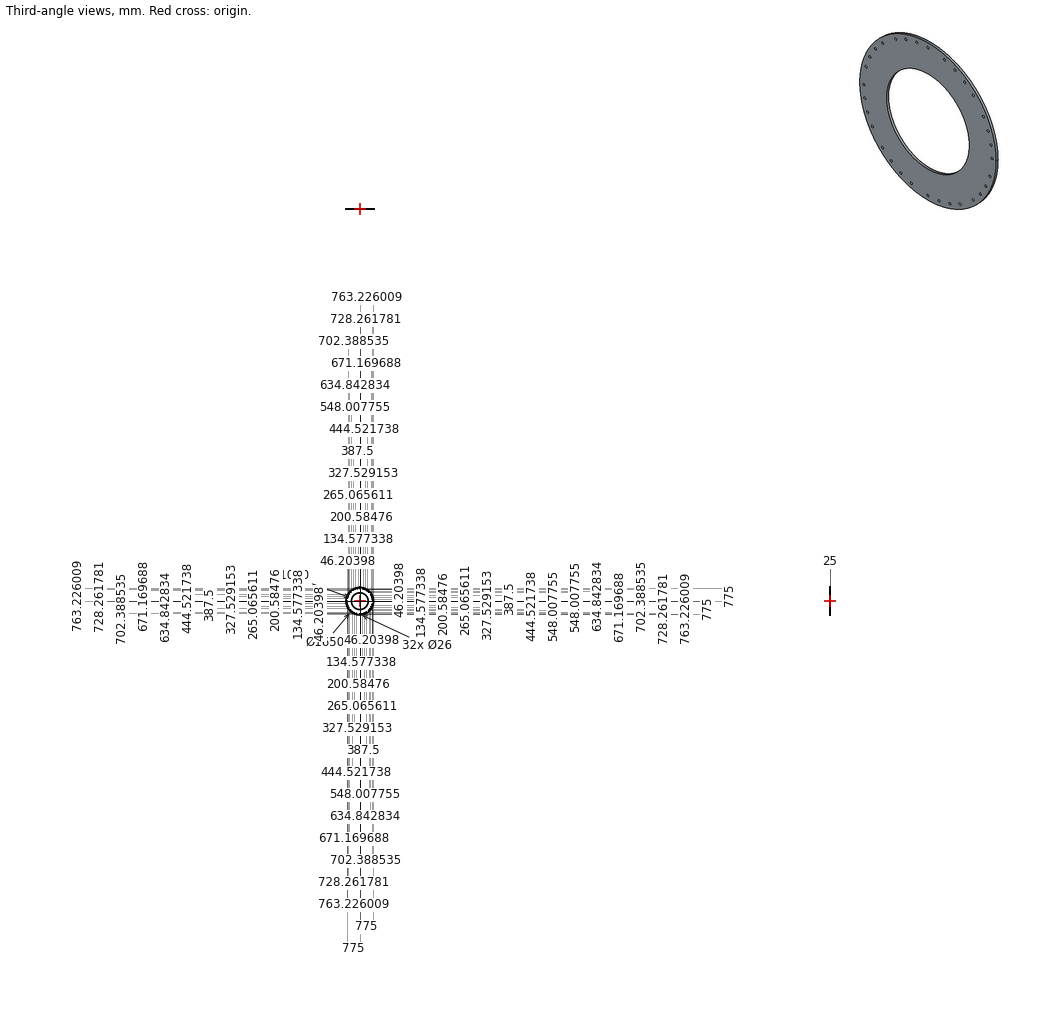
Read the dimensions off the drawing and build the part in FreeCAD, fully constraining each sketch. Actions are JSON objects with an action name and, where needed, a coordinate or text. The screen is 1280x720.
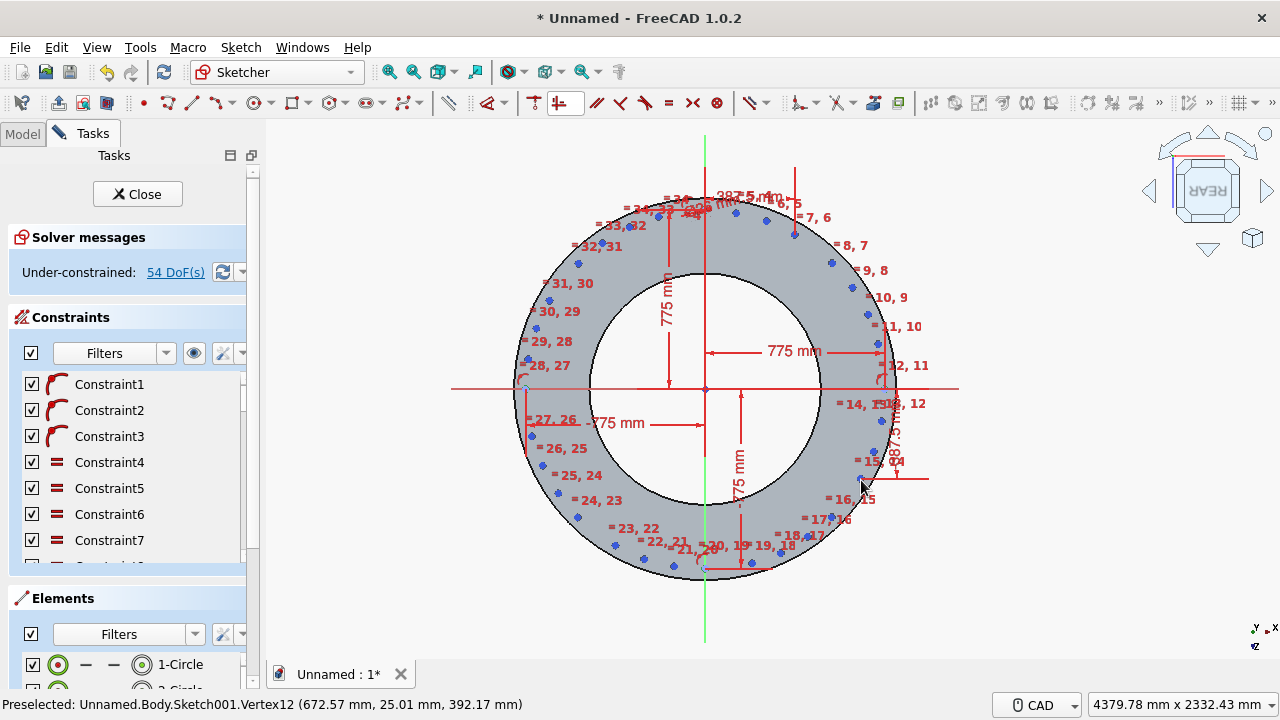
{"action": "left_click", "coordinate": [615, 546]}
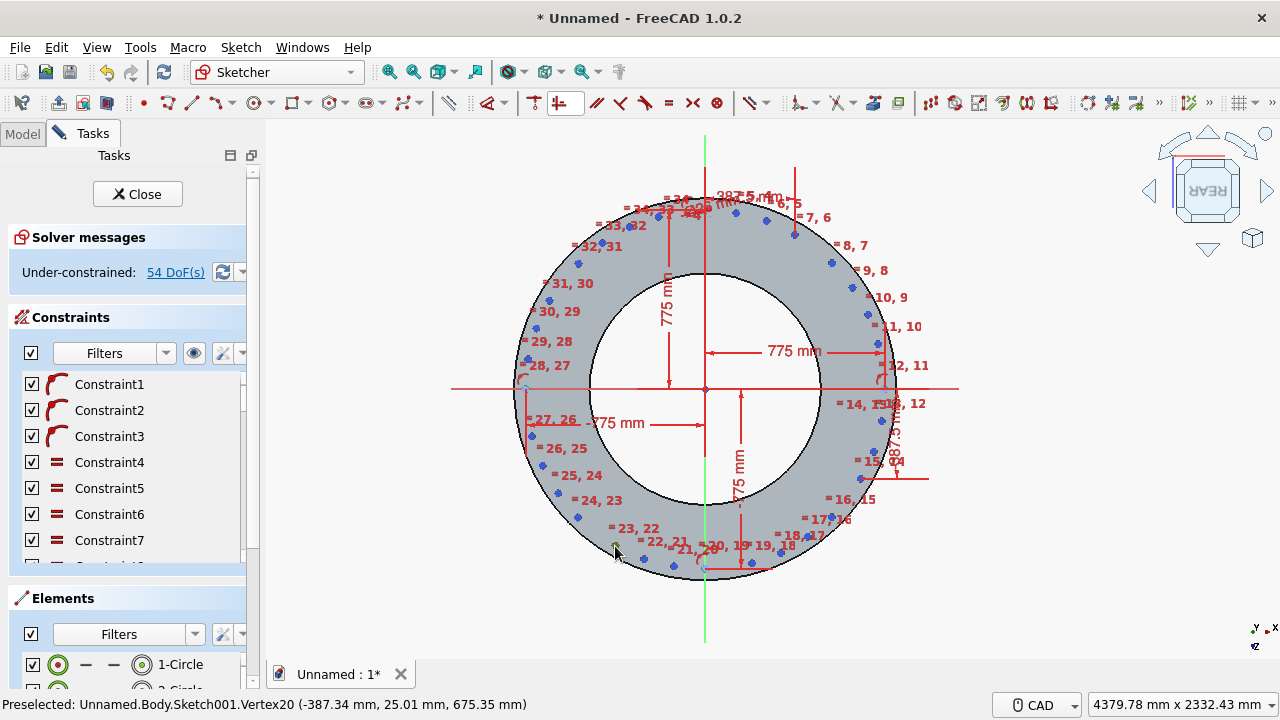
{"action": "left_click", "coordinate": [506, 104]}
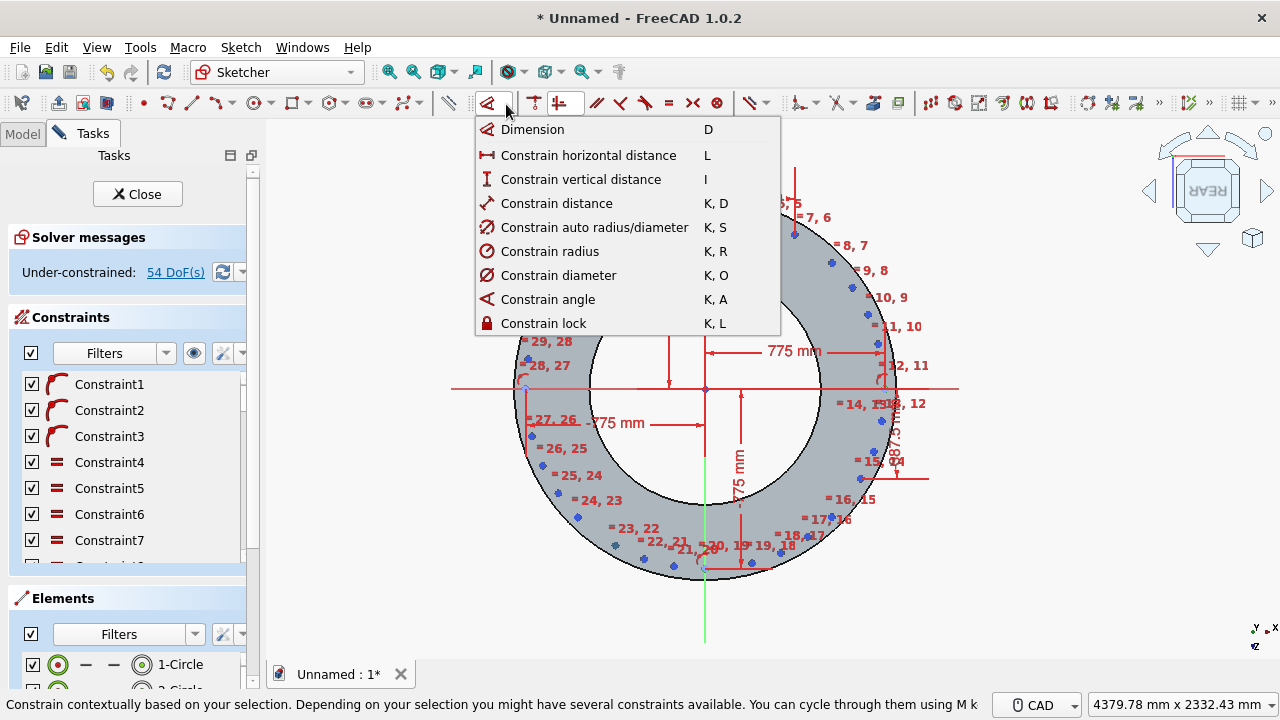
{"action": "left_click", "coordinate": [628, 155]}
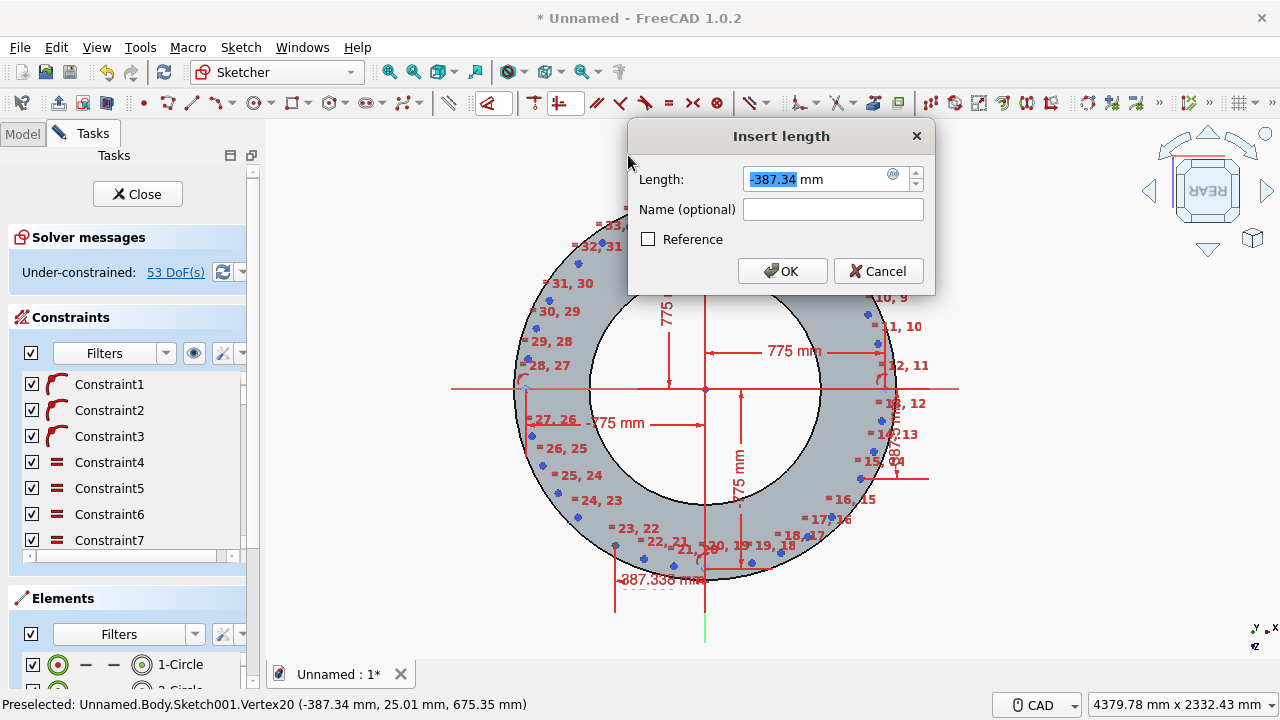
{"action": "type", "text": "-387.5"}
{"action": "key", "text": "Return"}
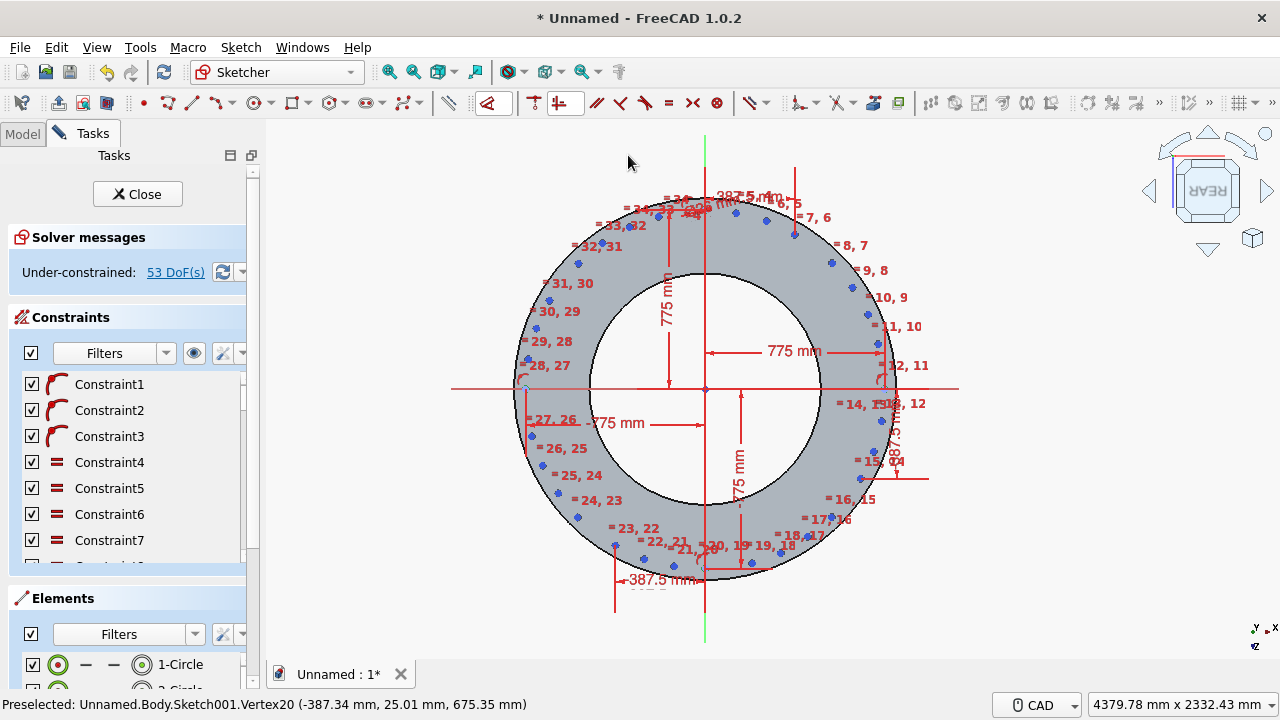
{"action": "left_click", "coordinate": [550, 301]}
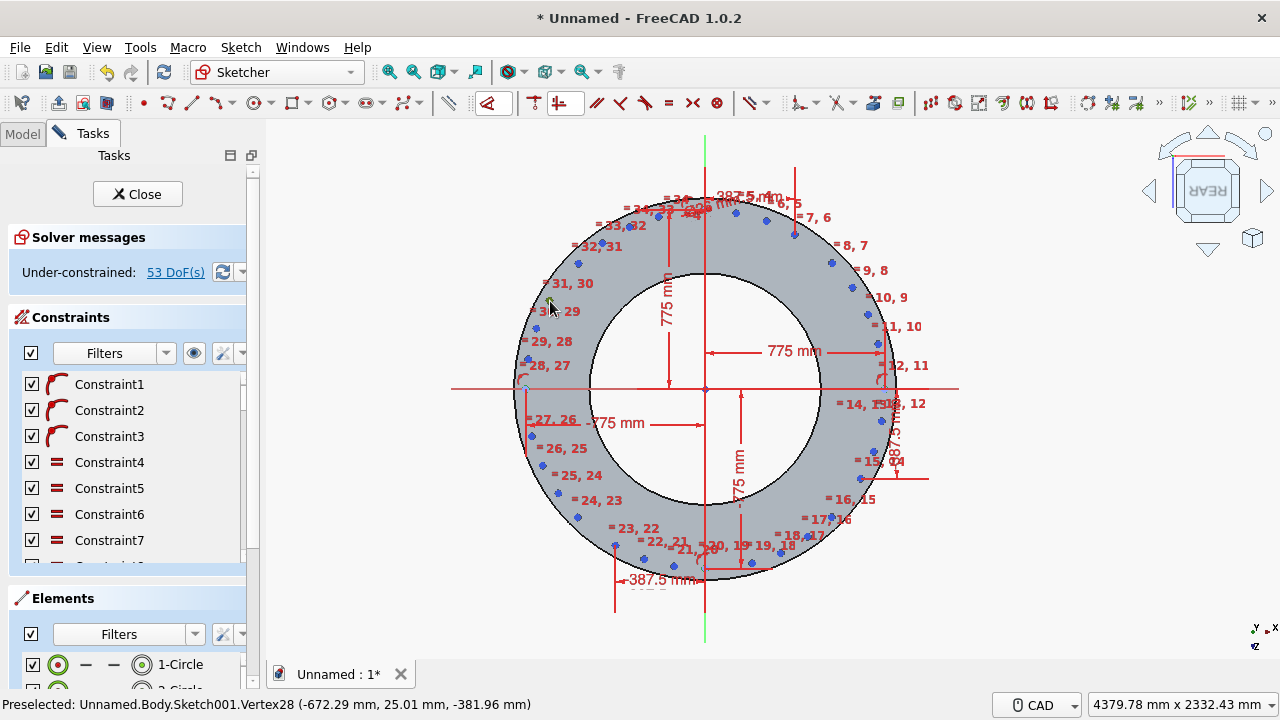
{"action": "key", "text": "i"}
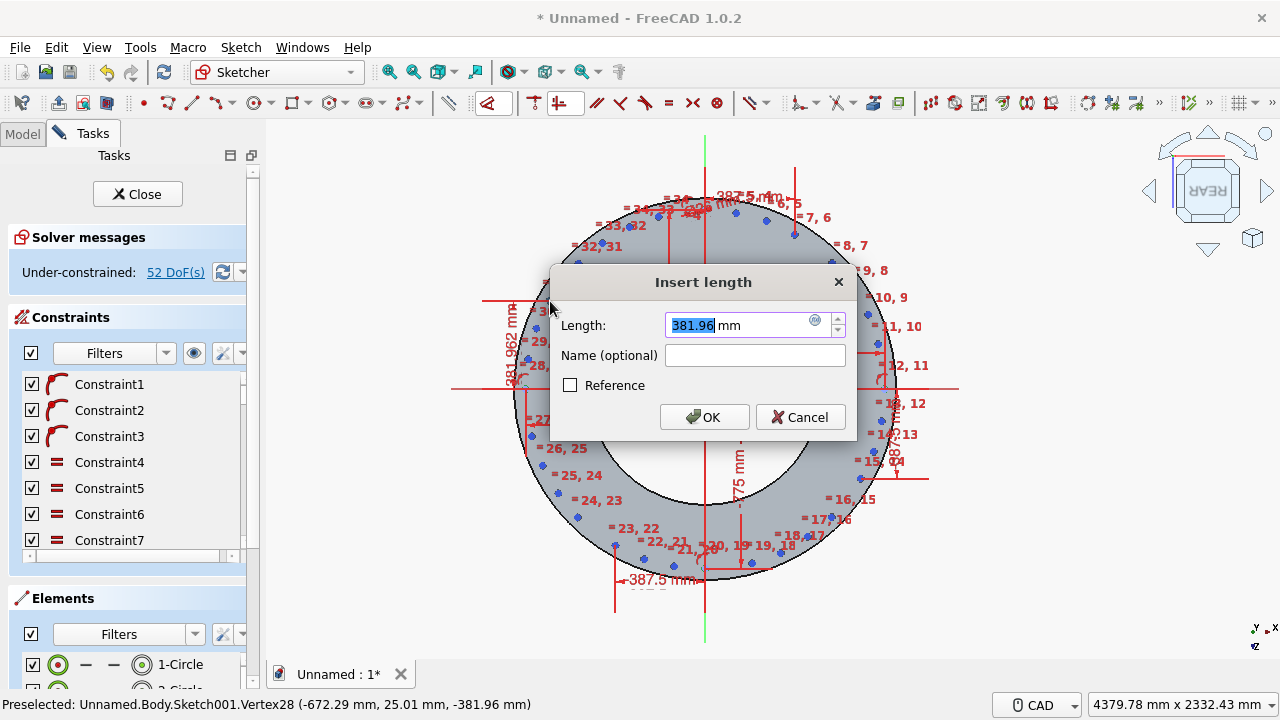
{"action": "type", "text": "387.5"}
{"action": "key", "text": "Return"}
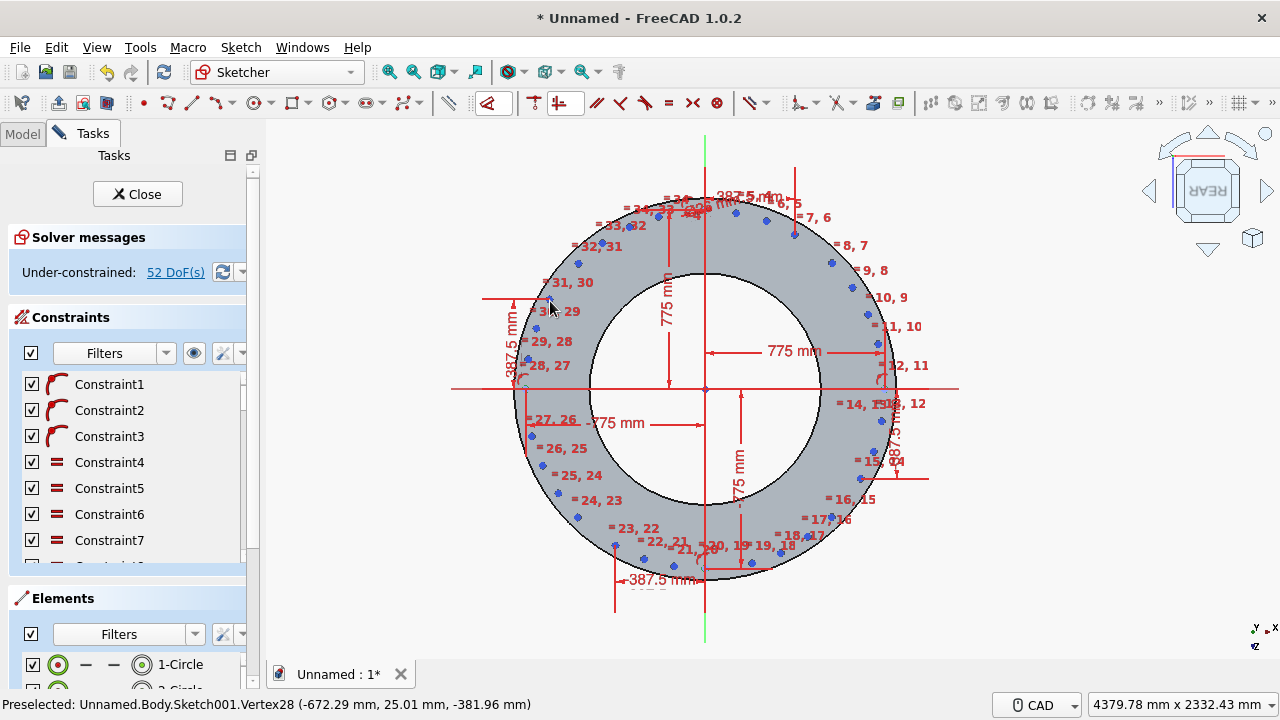
{"action": "left_click", "coordinate": [878, 344]}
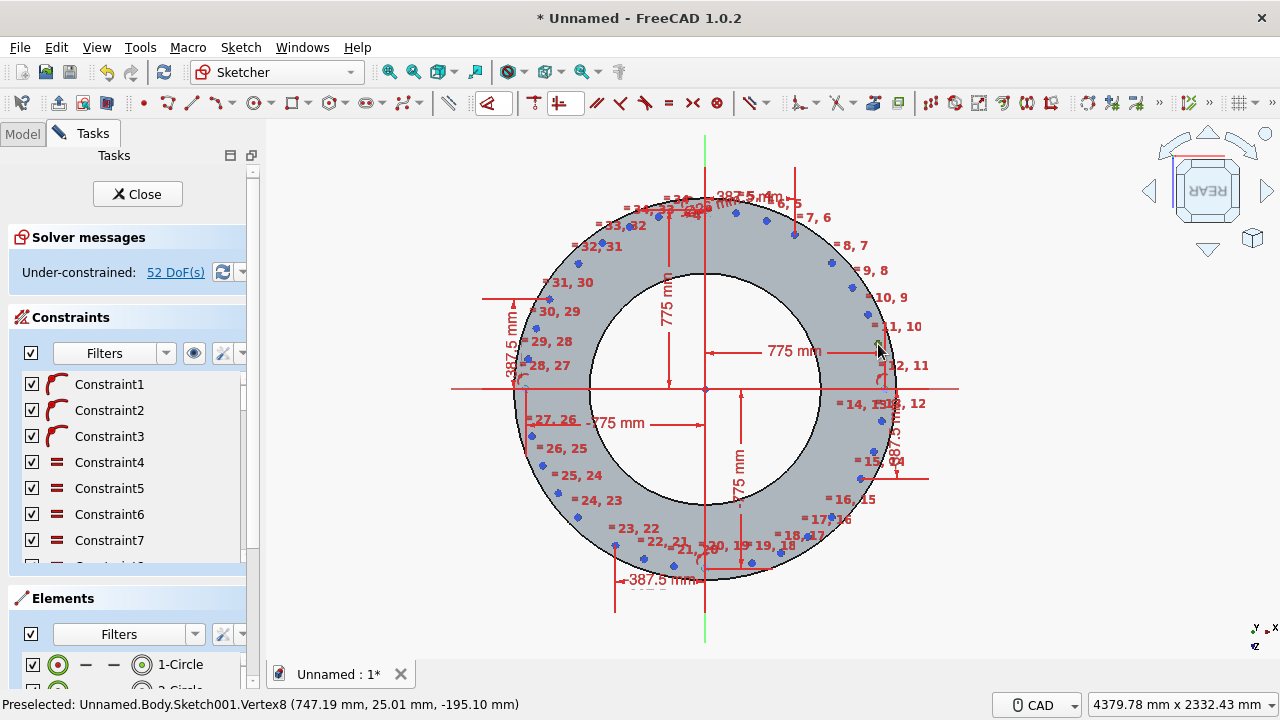
{"action": "key", "text": "i"}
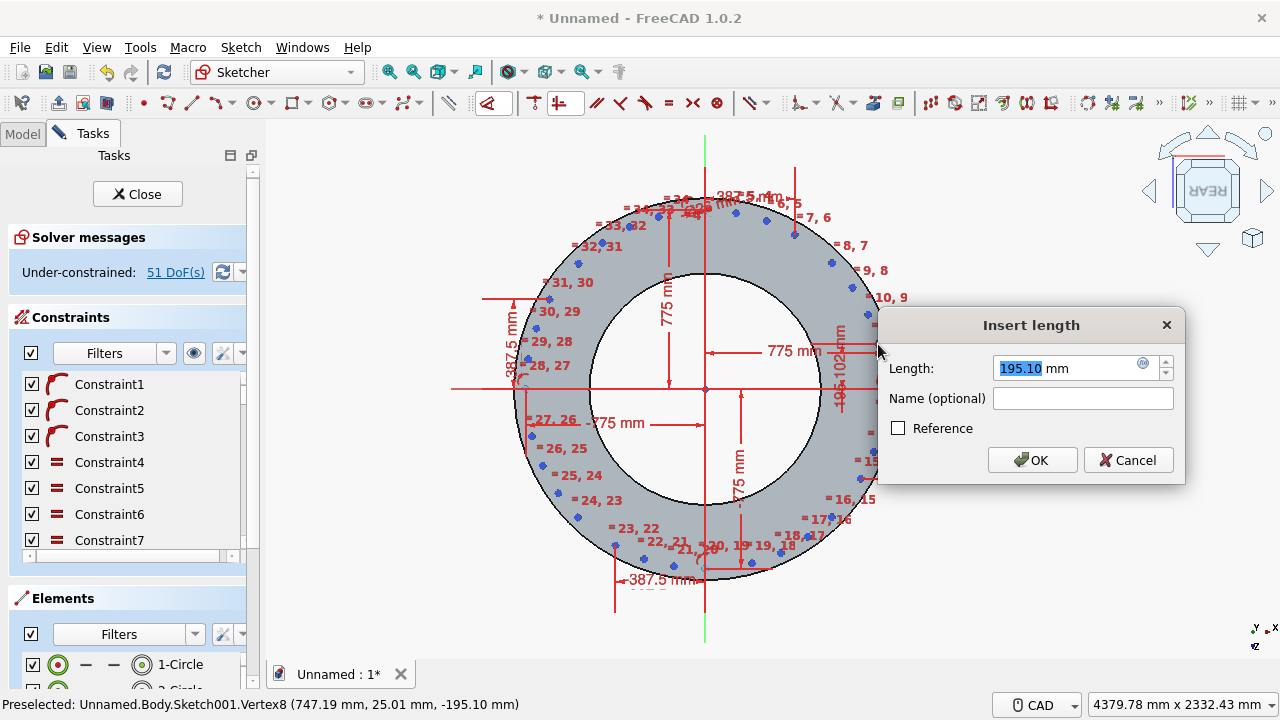
{"action": "type", "text": "200.58476"}
{"action": "key", "text": "Return"}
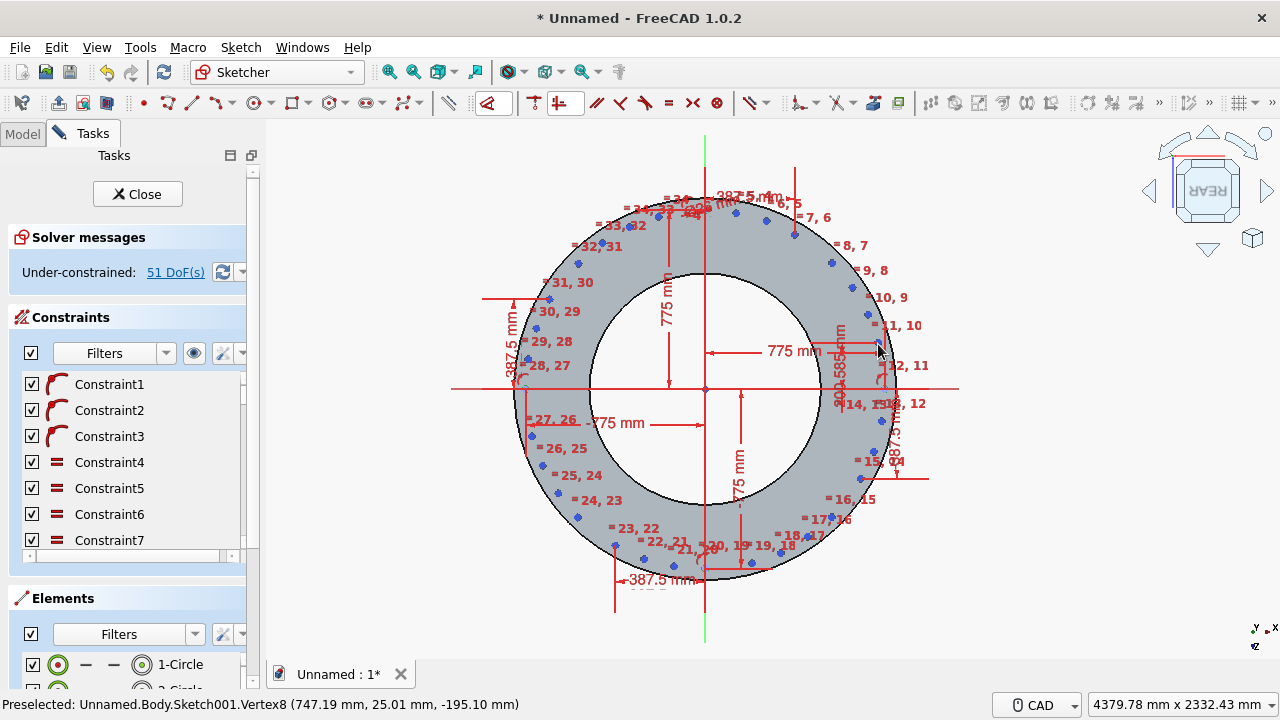
{"action": "left_click", "coordinate": [752, 563]}